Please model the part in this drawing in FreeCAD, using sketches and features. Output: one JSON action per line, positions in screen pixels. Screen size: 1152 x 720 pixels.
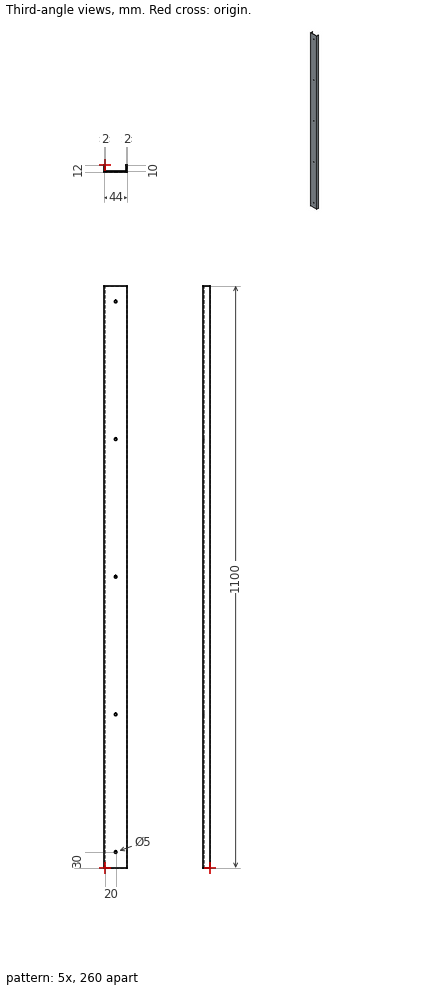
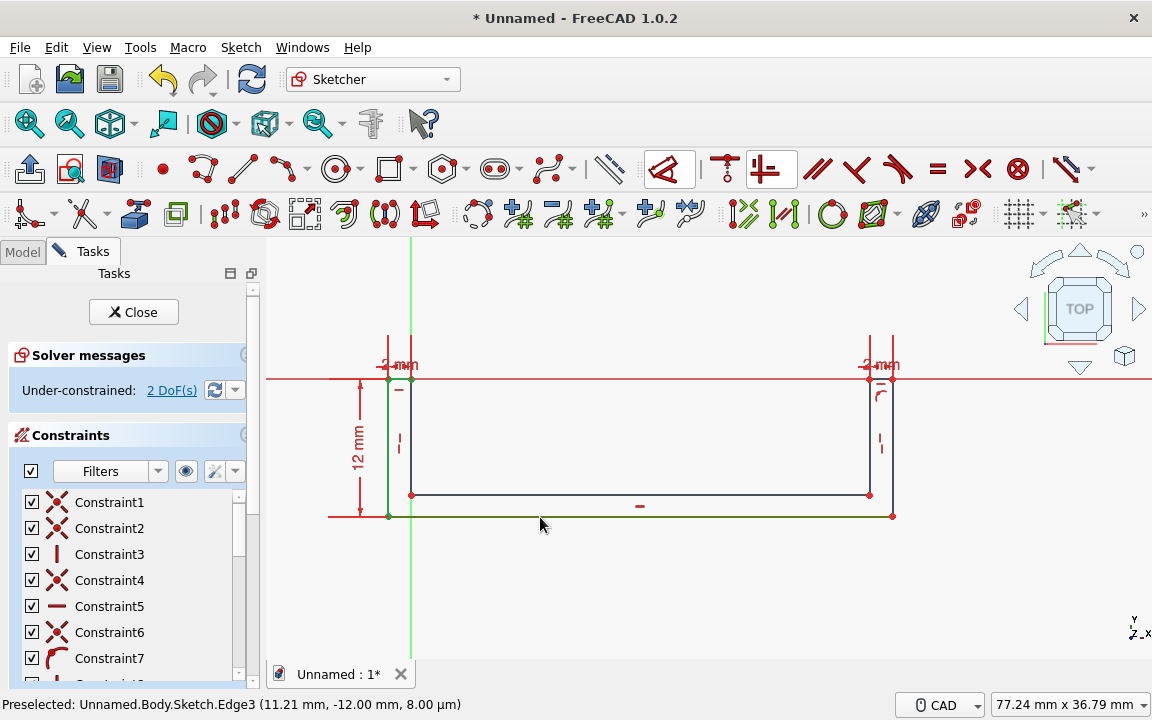
{"action": "left_click", "coordinate": [690, 170]}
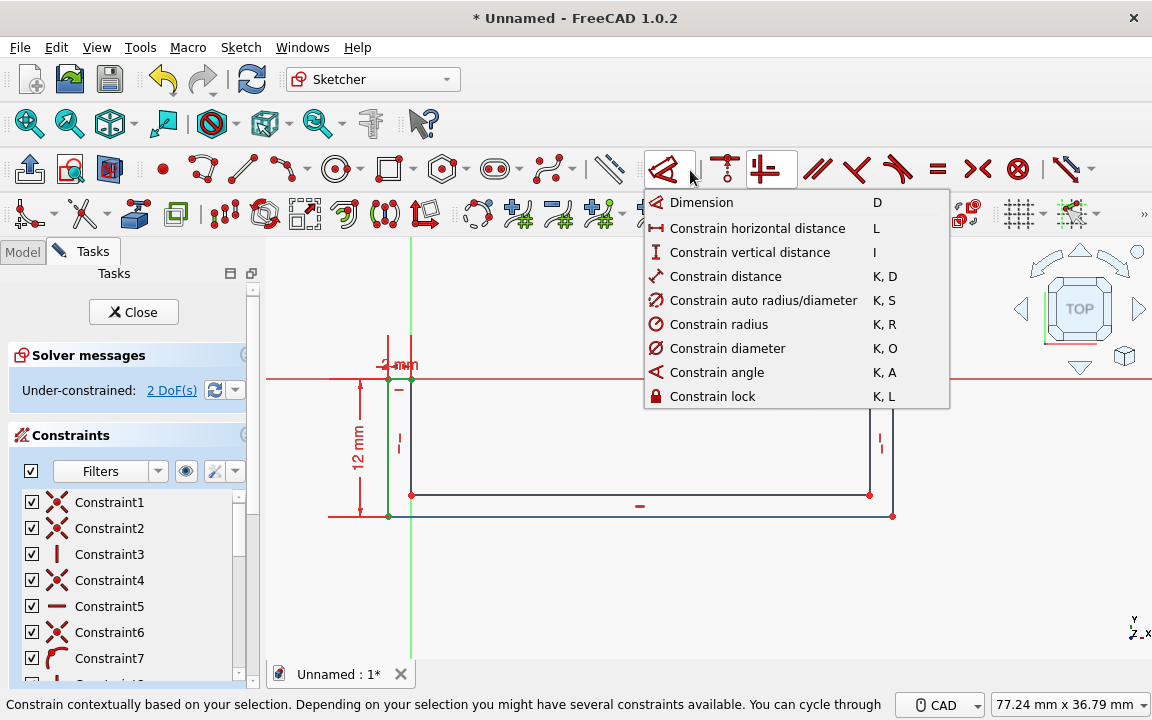
{"action": "left_click", "coordinate": [797, 228]}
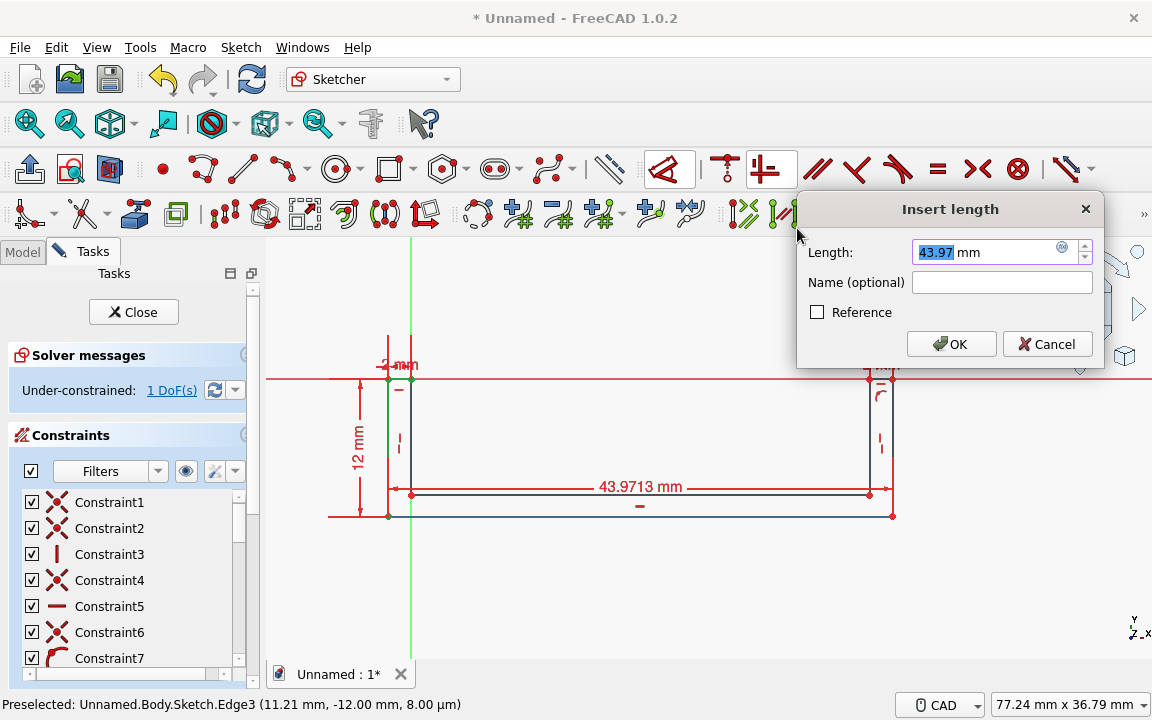
{"action": "type", "text": "44"}
{"action": "key", "text": "Return"}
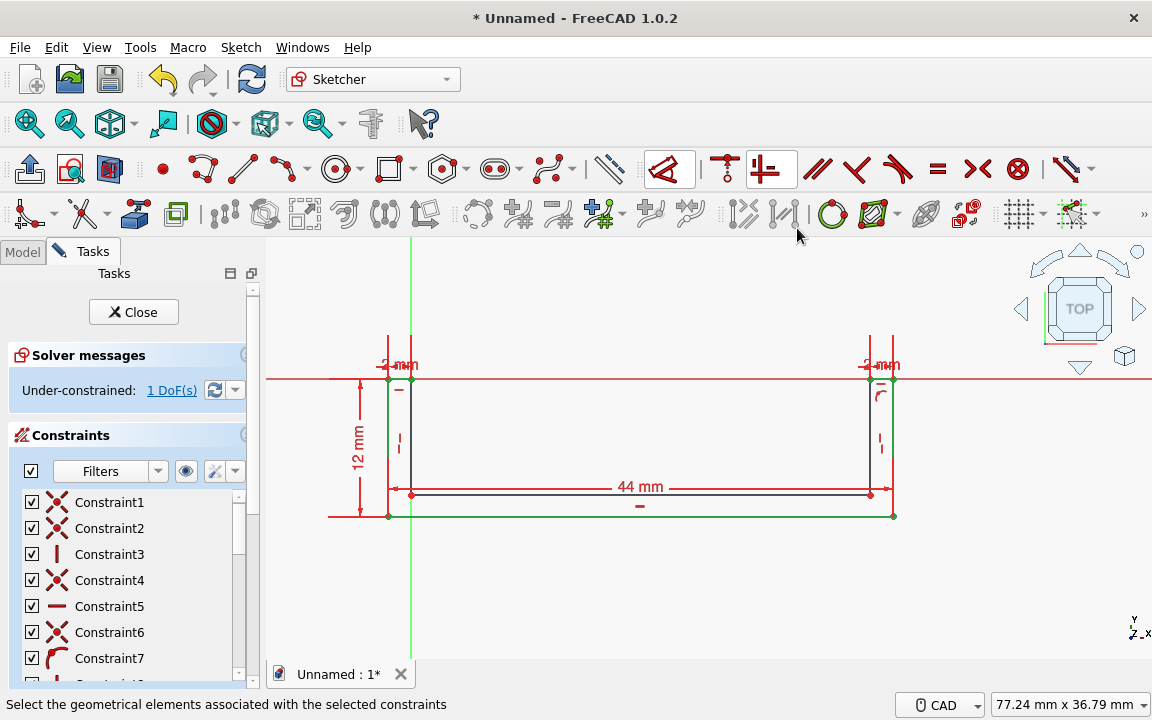
{"action": "left_click", "coordinate": [870, 414]}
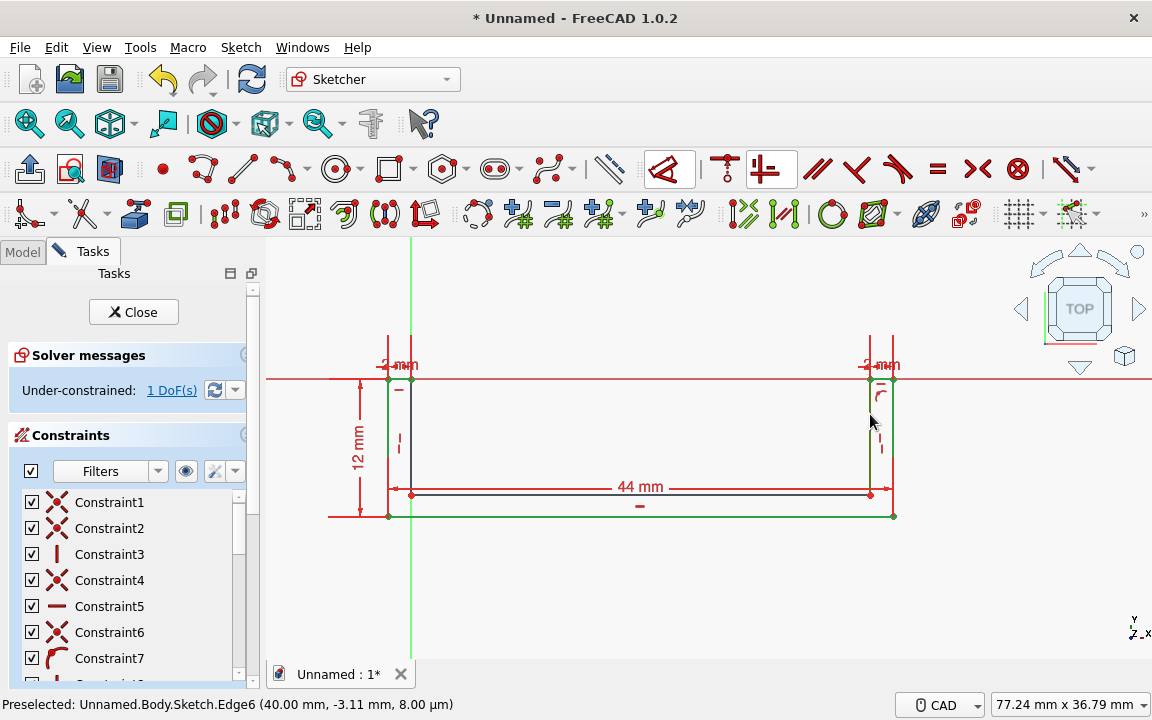
{"action": "left_click", "coordinate": [690, 170]}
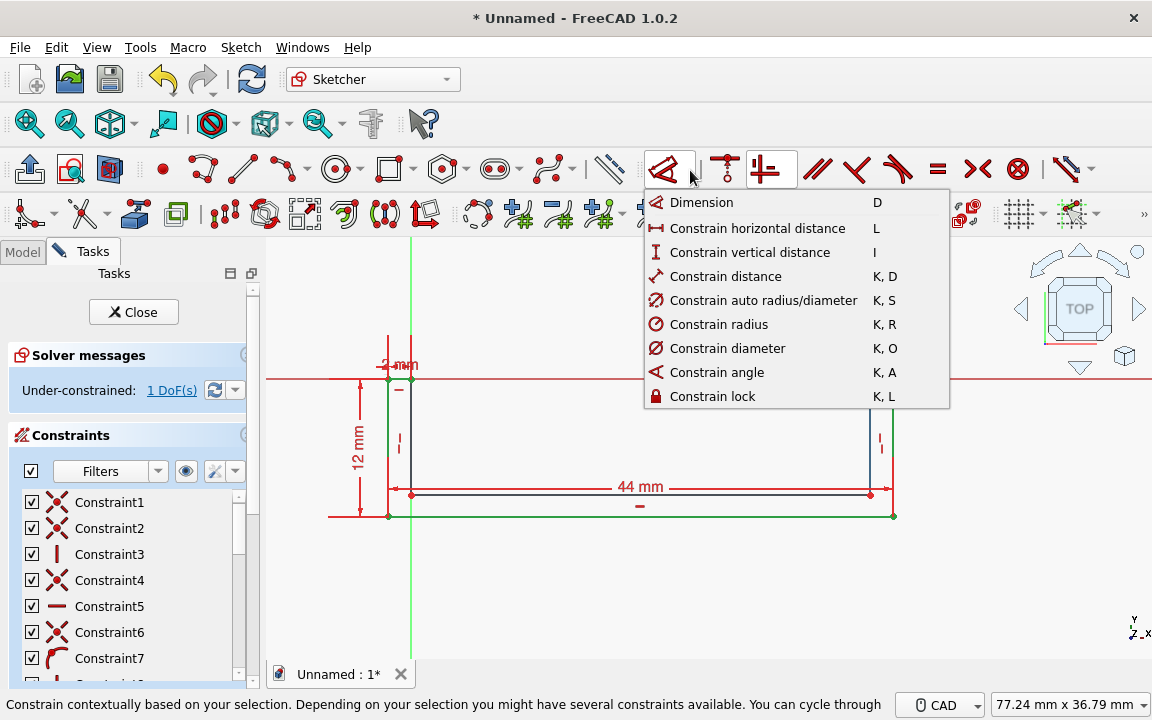
{"action": "left_click", "coordinate": [797, 252]}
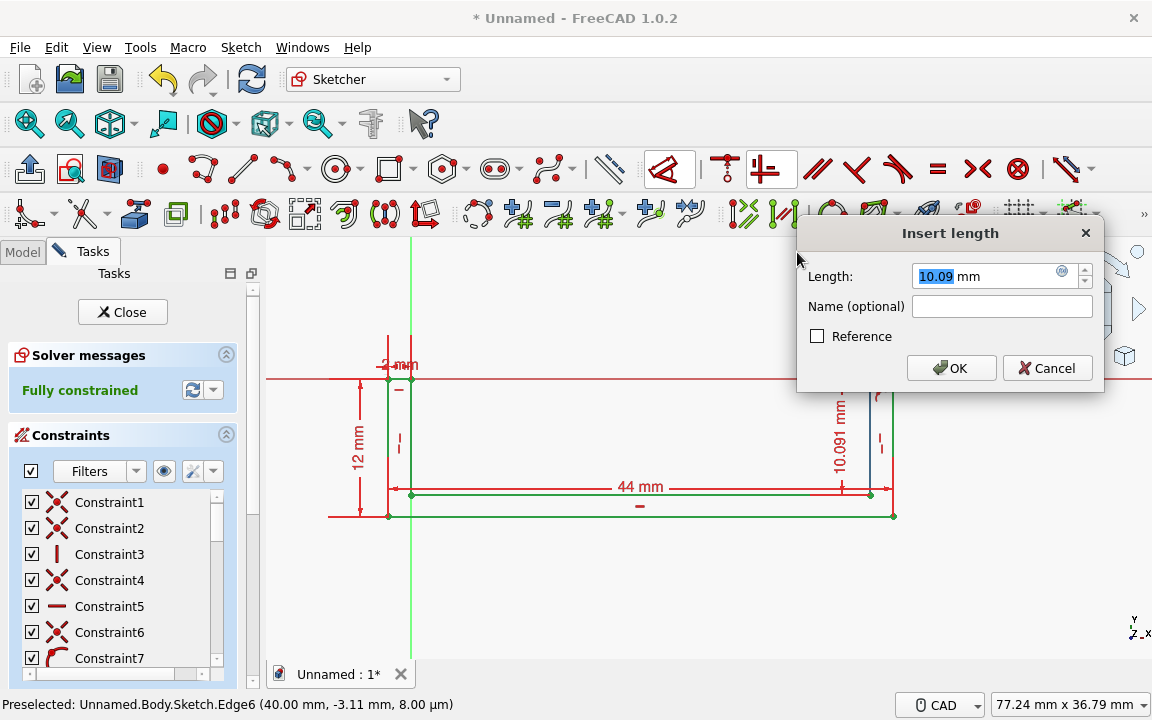
{"action": "type", "text": "10"}
{"action": "key", "text": "Return"}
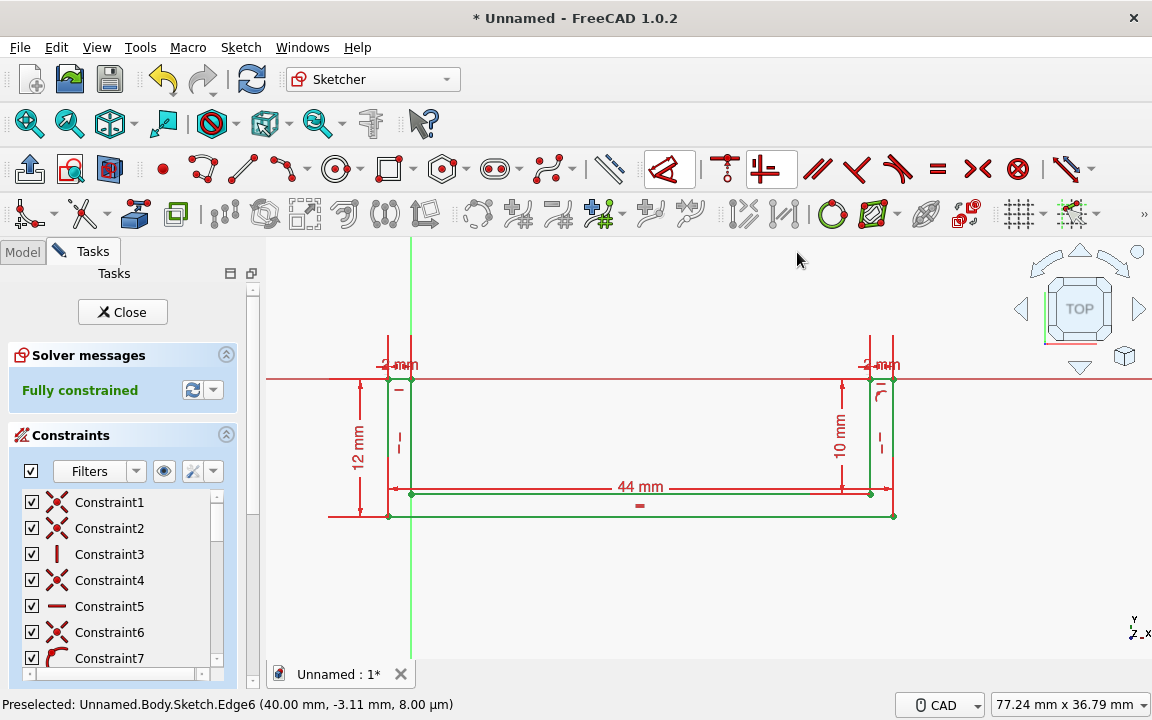
{"action": "left_click", "coordinate": [123, 312]}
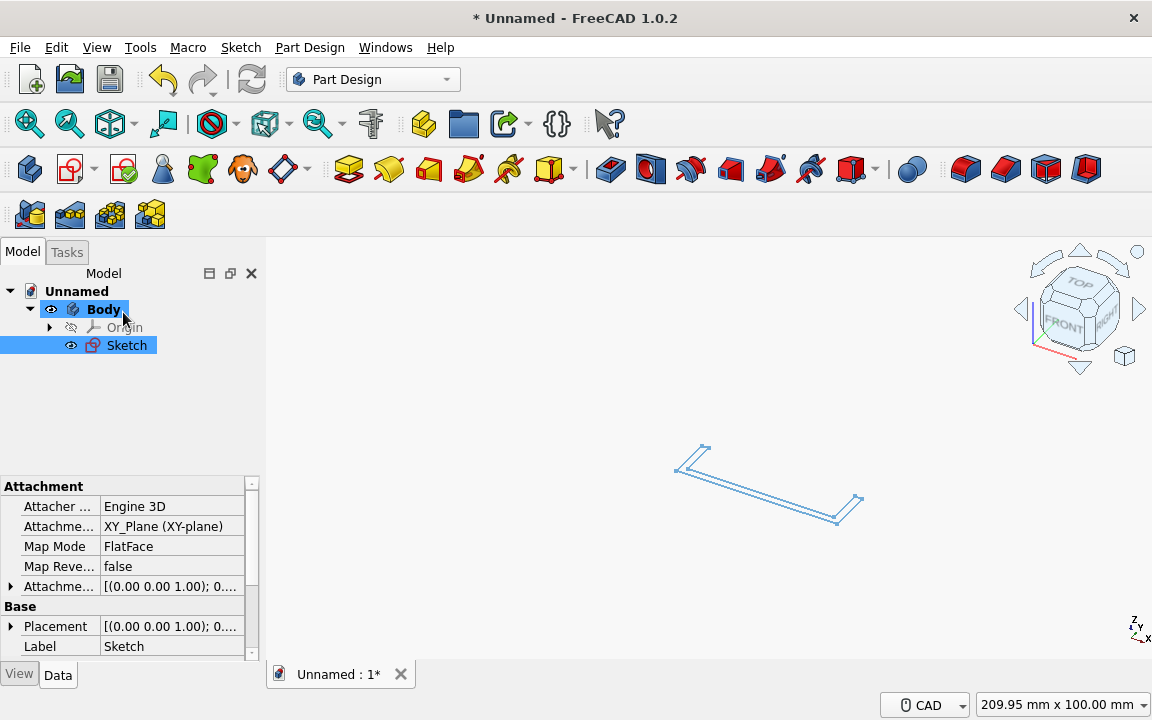
{"action": "left_click", "coordinate": [350, 170]}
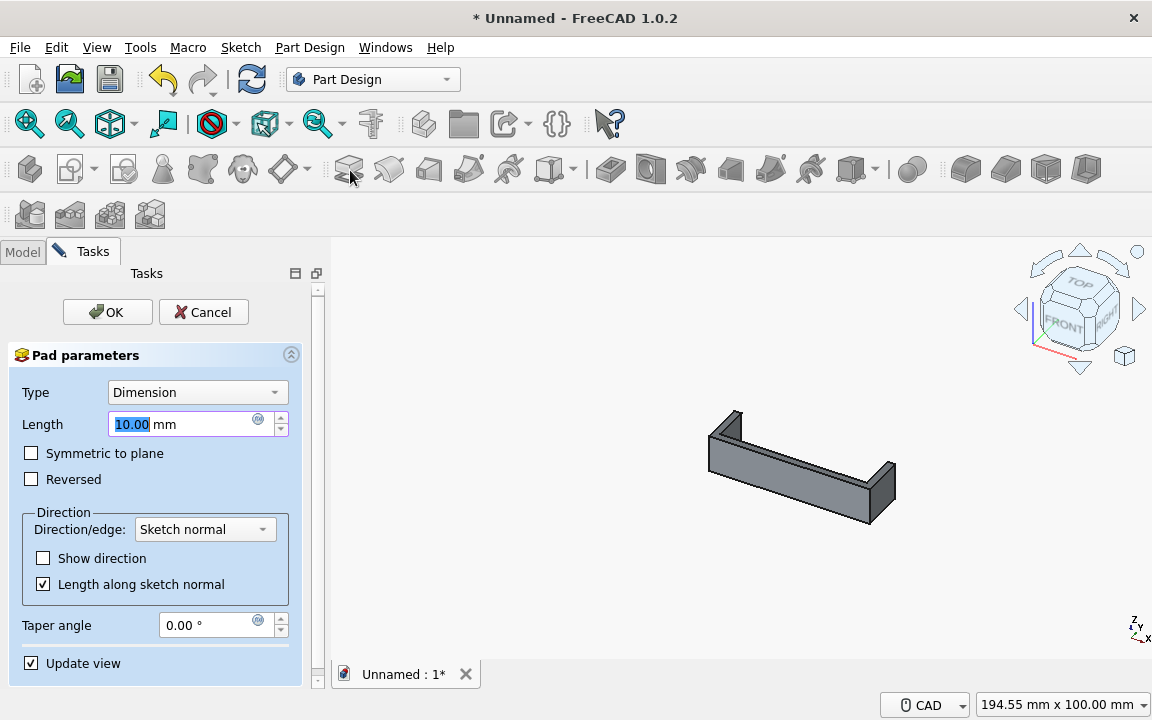
{"action": "type", "text": "1100"}
{"action": "key", "text": "Tab"}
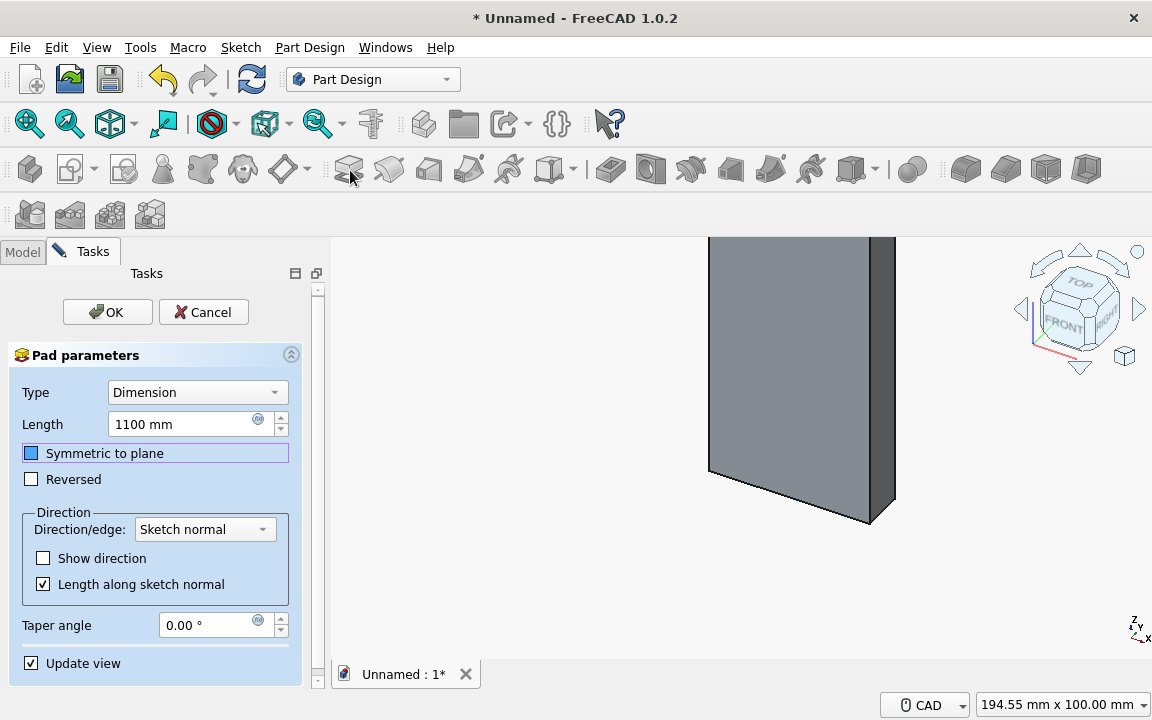
{"action": "left_click", "coordinate": [108, 312]}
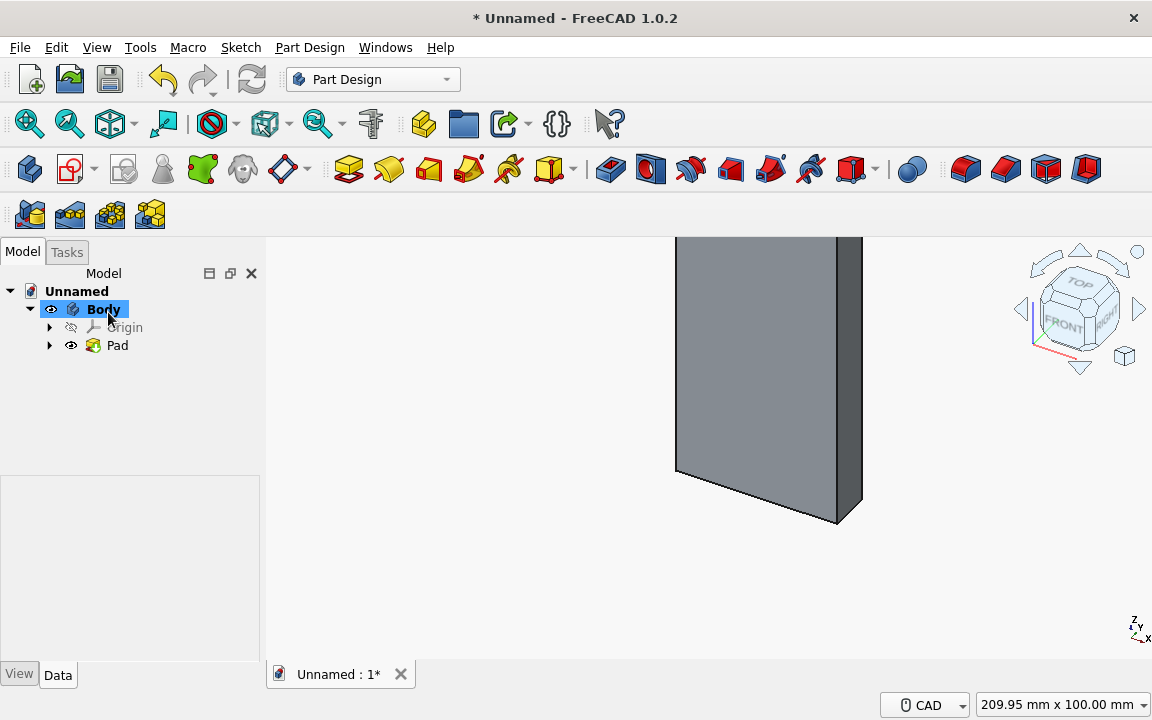
{"action": "left_click", "coordinate": [30, 124]}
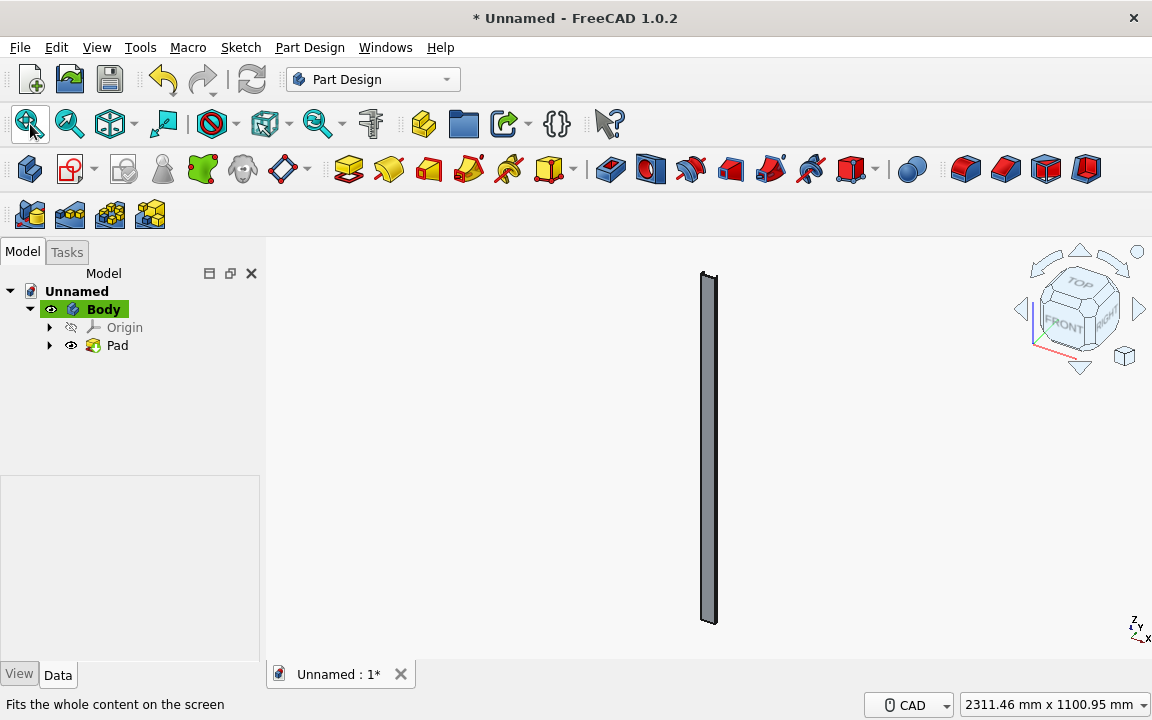
{"action": "key", "text": "4"}